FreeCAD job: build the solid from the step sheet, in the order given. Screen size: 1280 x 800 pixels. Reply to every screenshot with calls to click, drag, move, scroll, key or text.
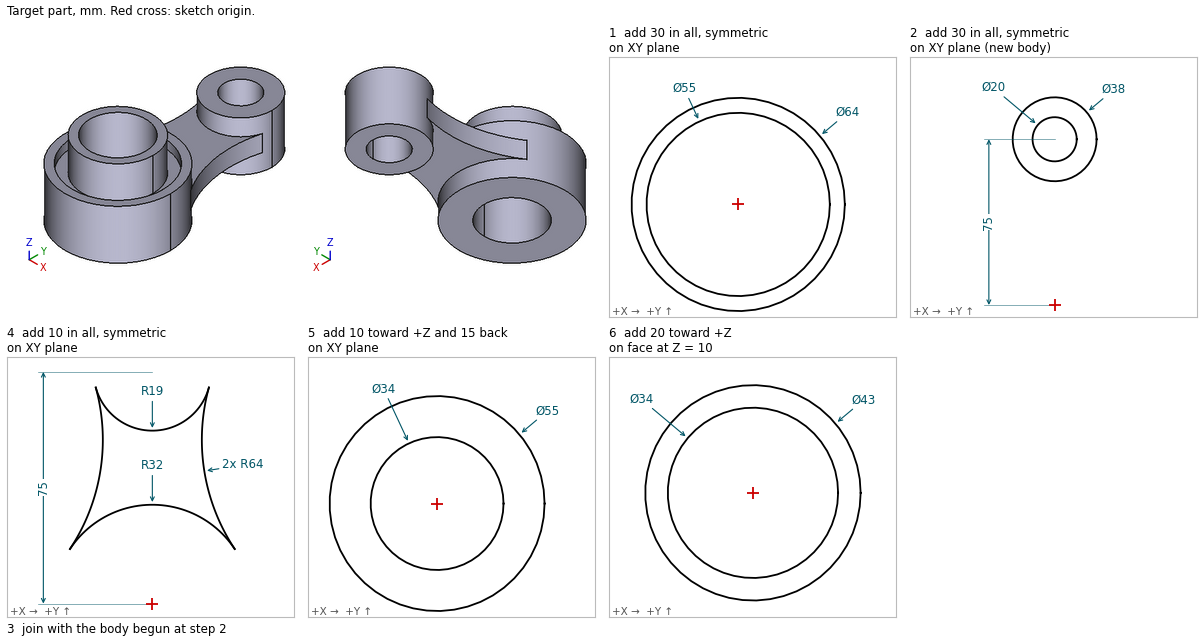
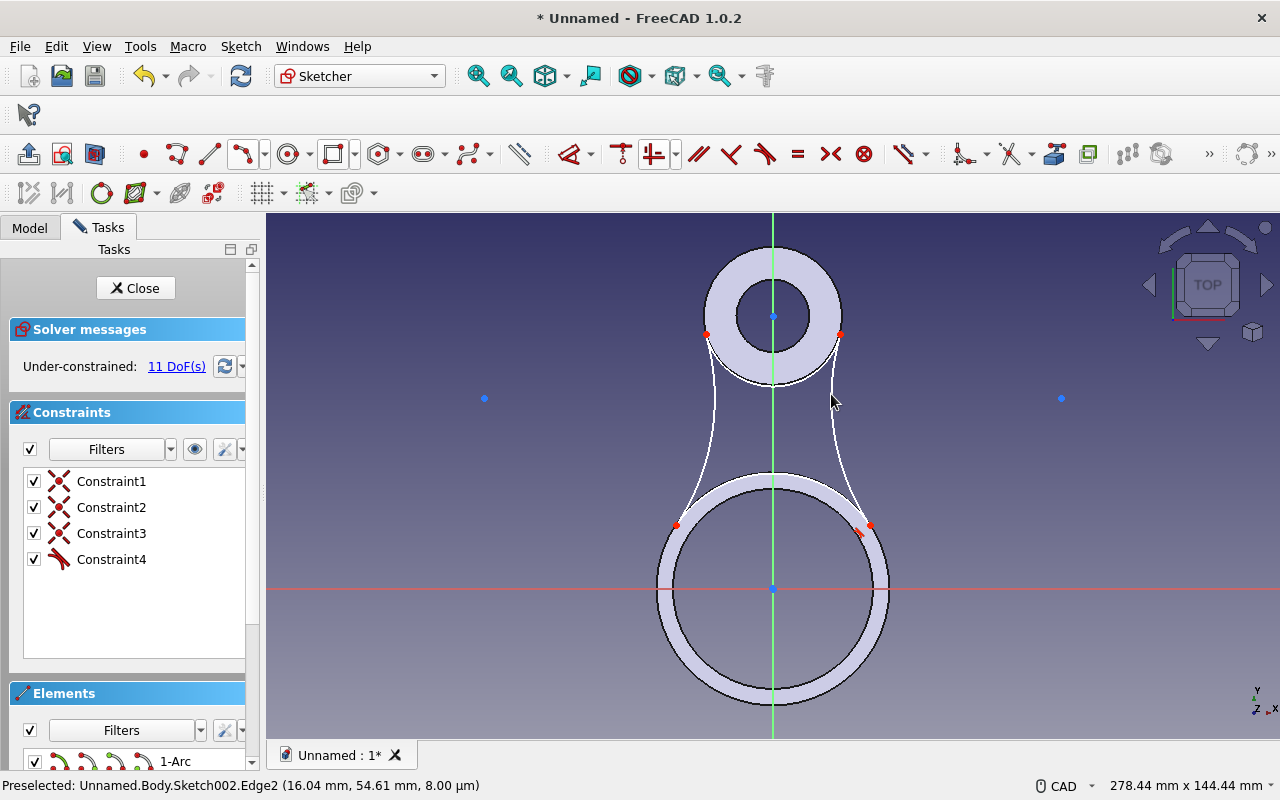
click(818, 482)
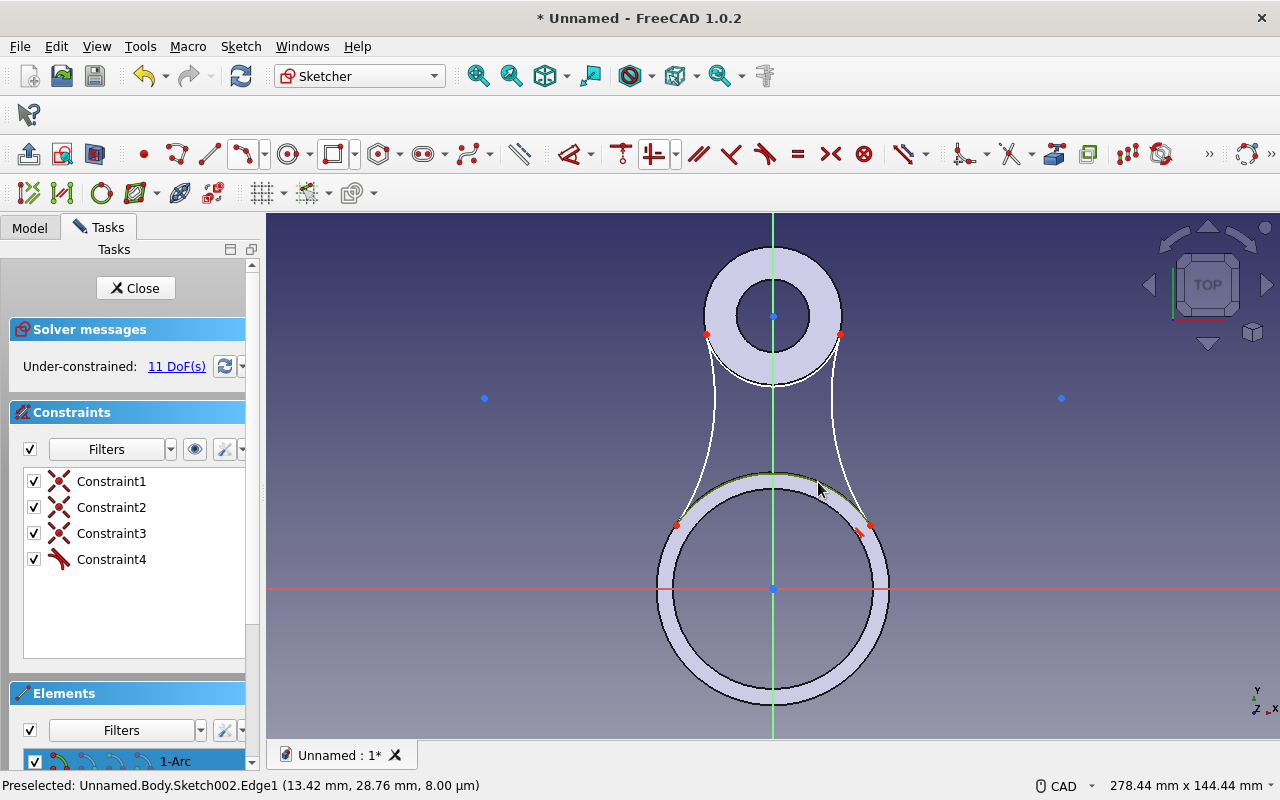
click(702, 472)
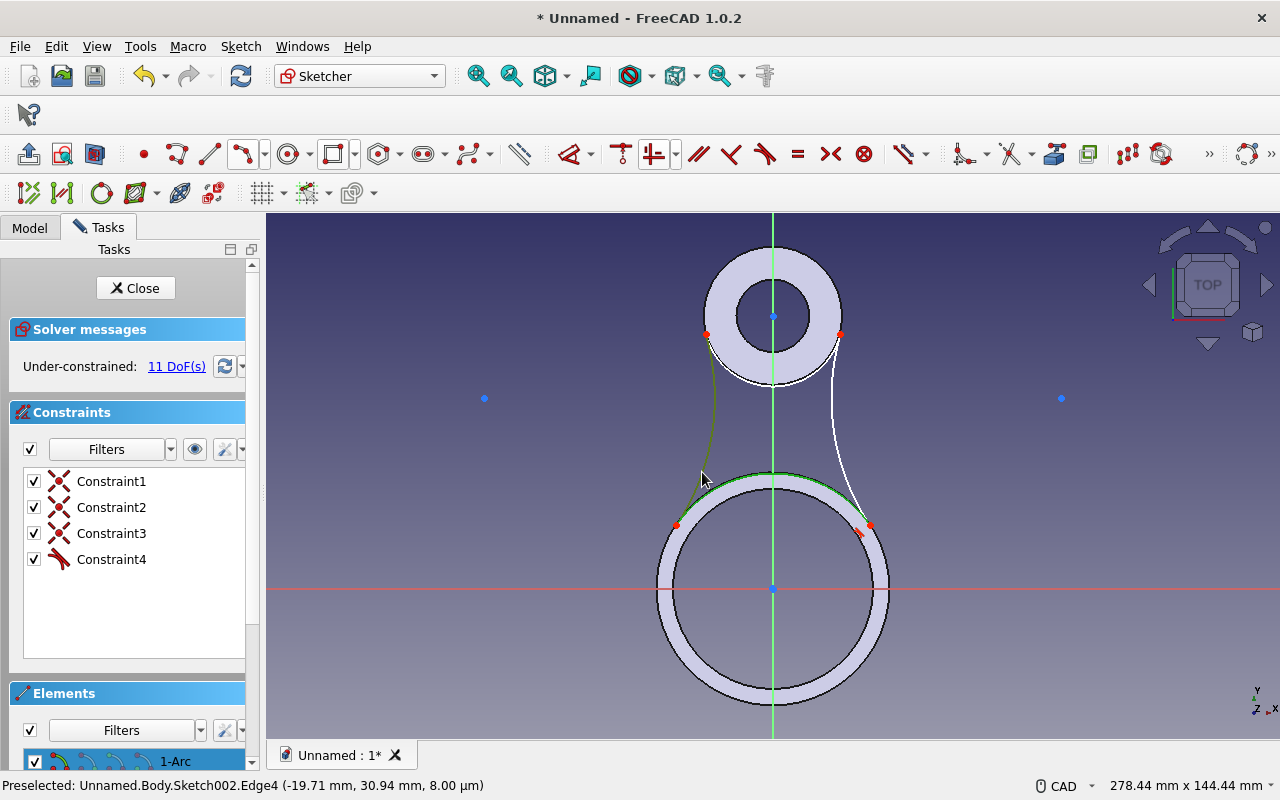
click(765, 154)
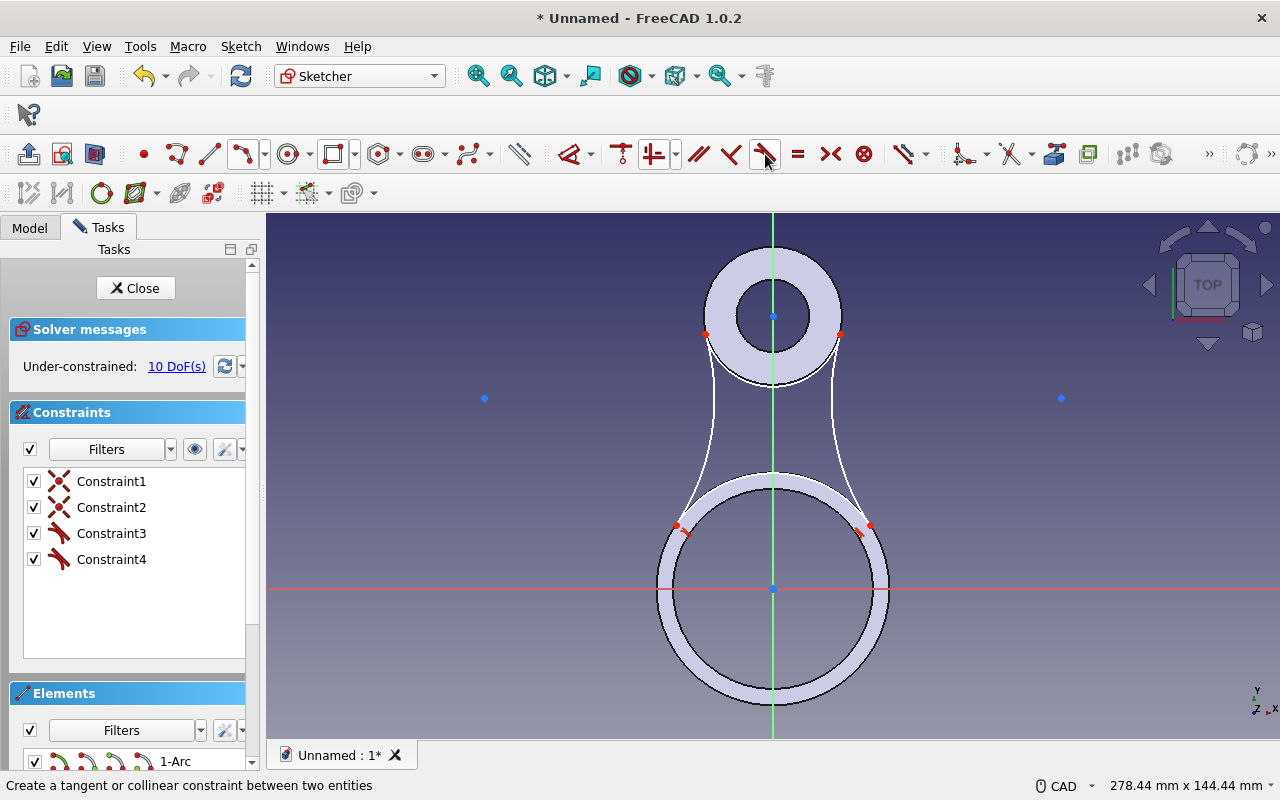
click(832, 394)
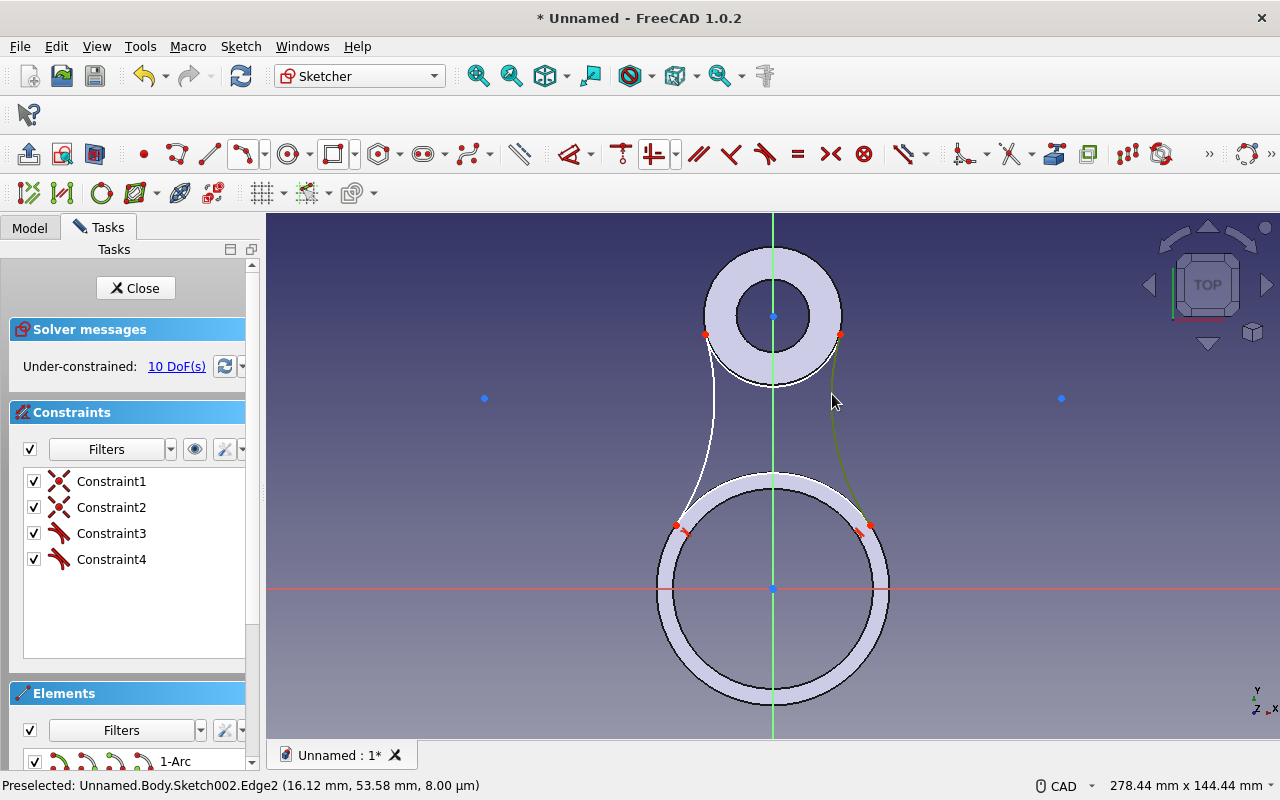
click(738, 377)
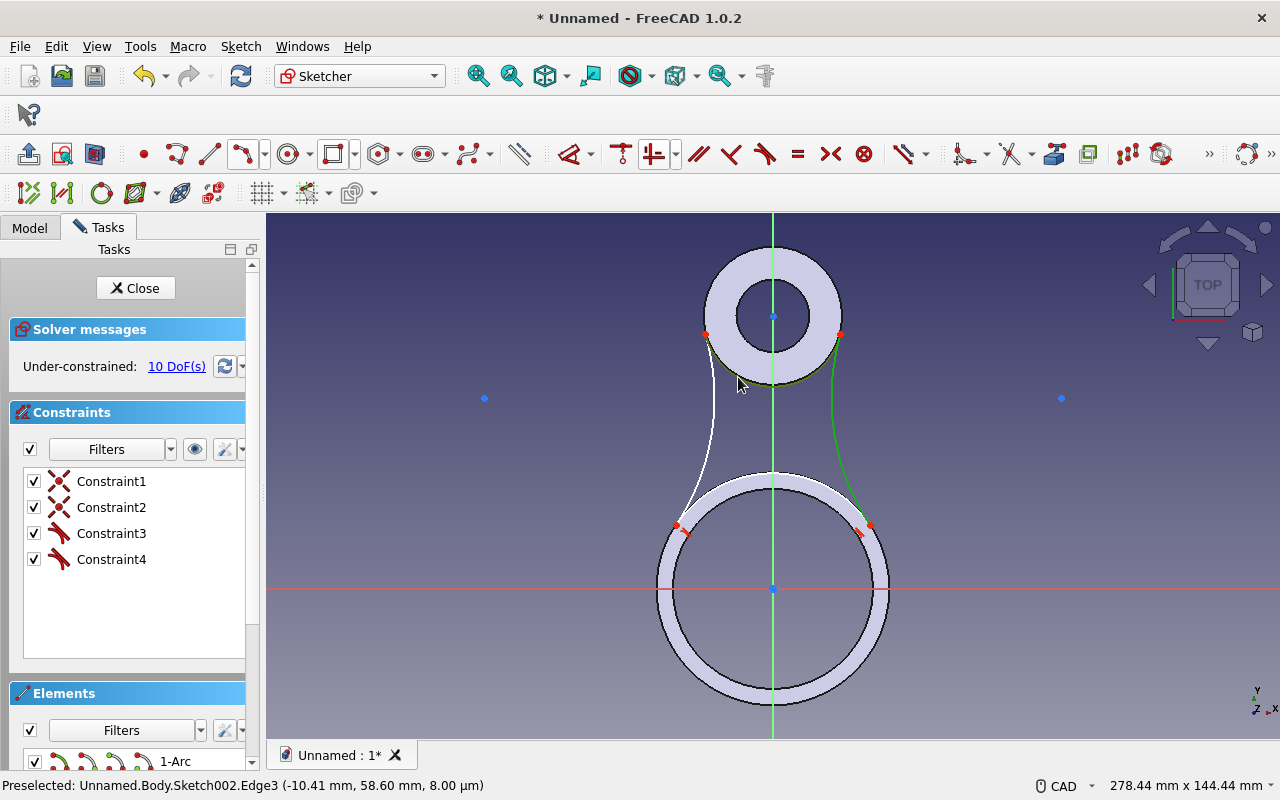
key(t)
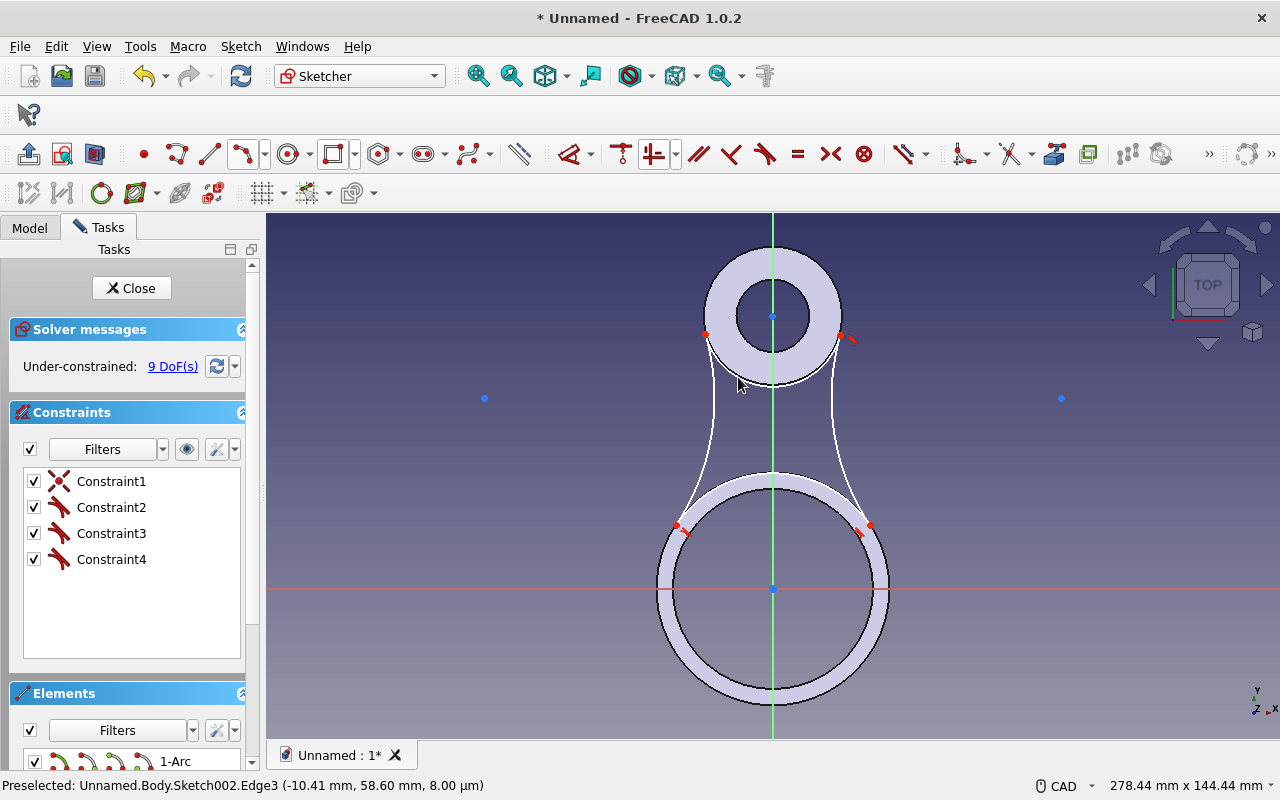
click(738, 377)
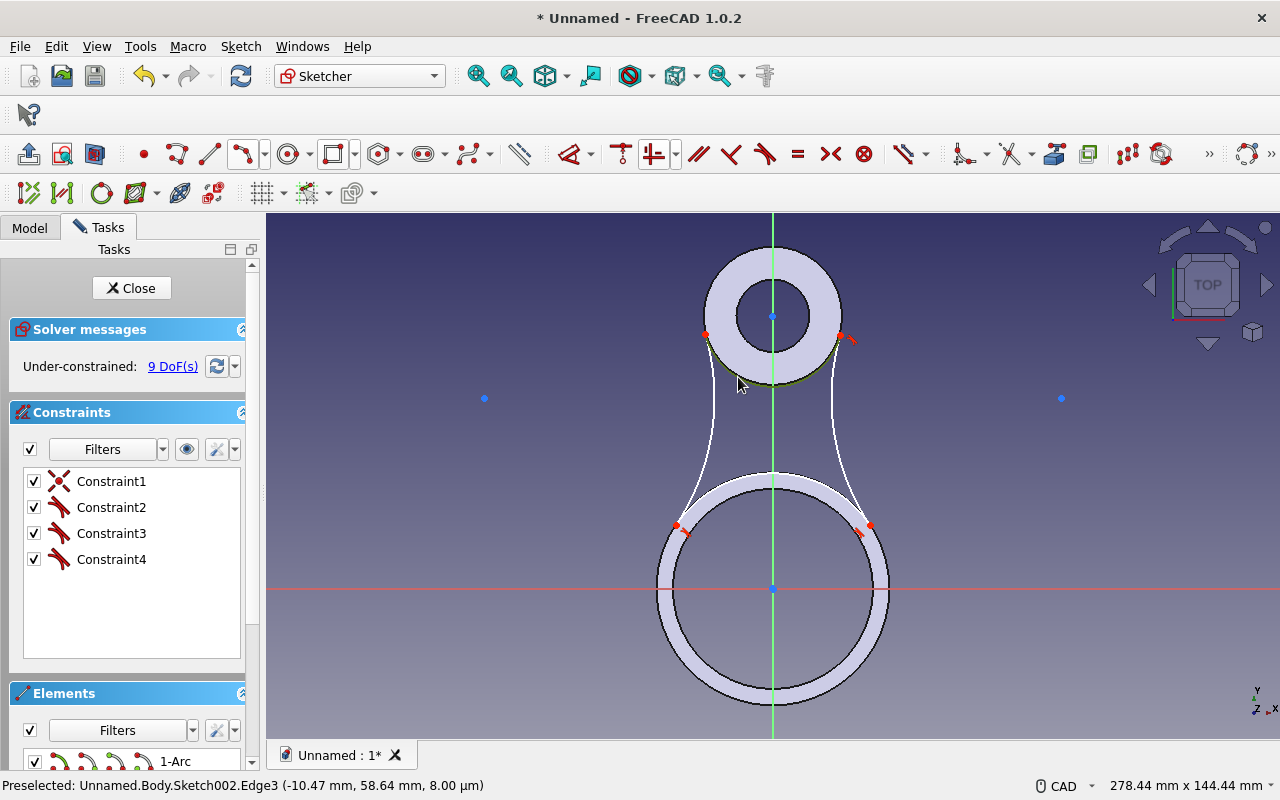
click(702, 472)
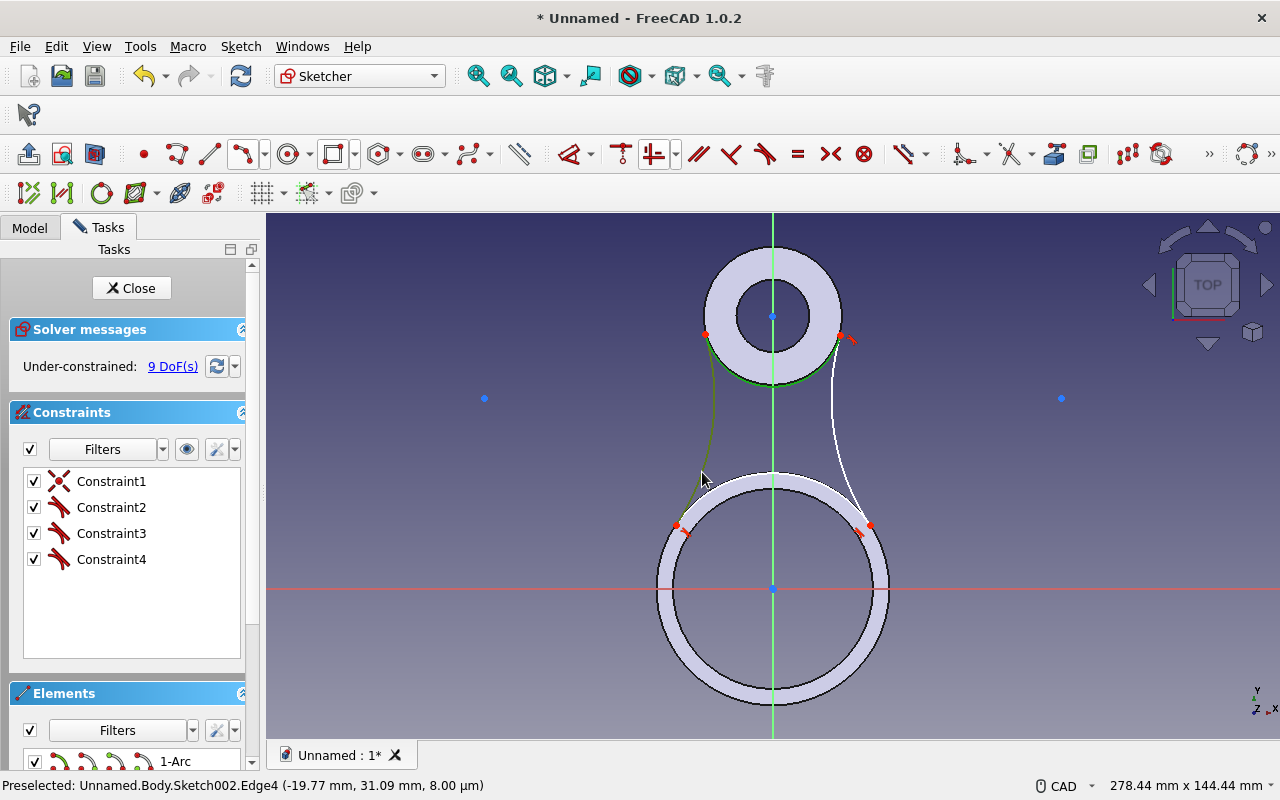
key(t)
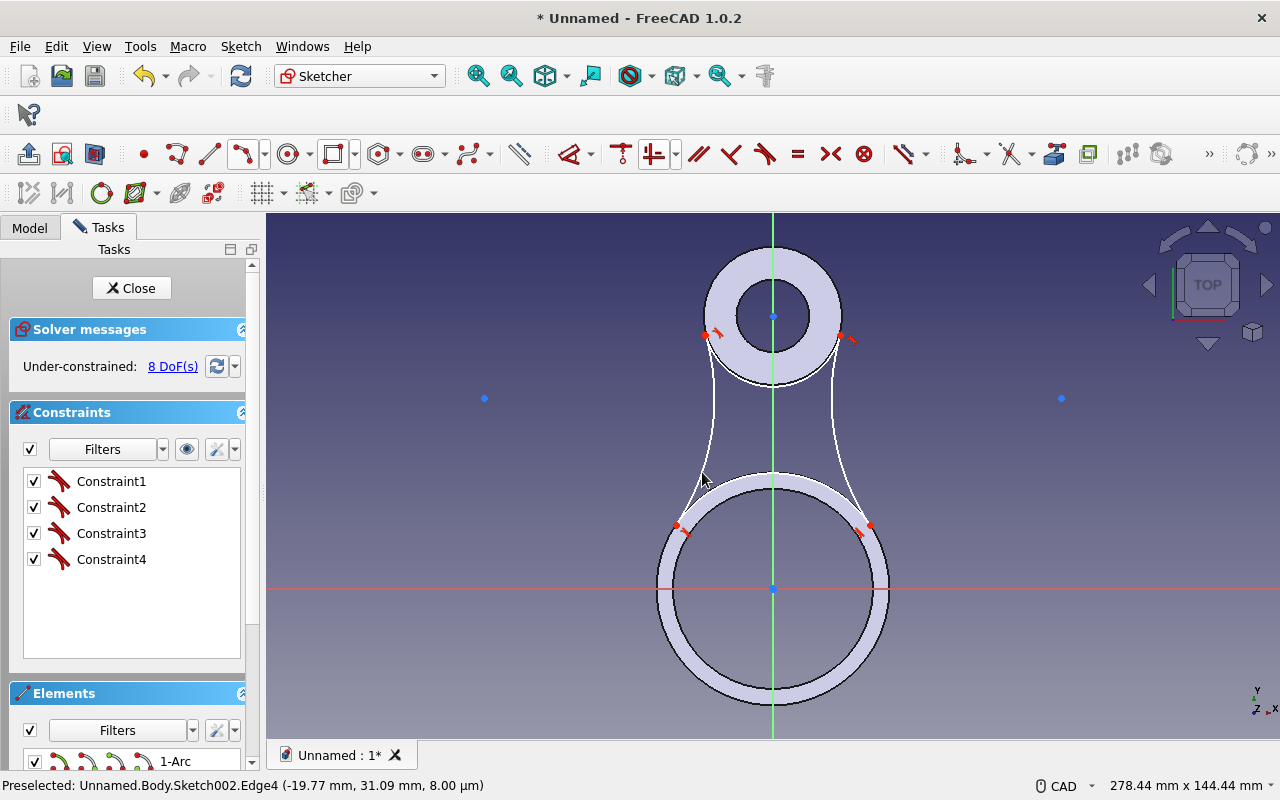
drag(763, 579, 783, 600)